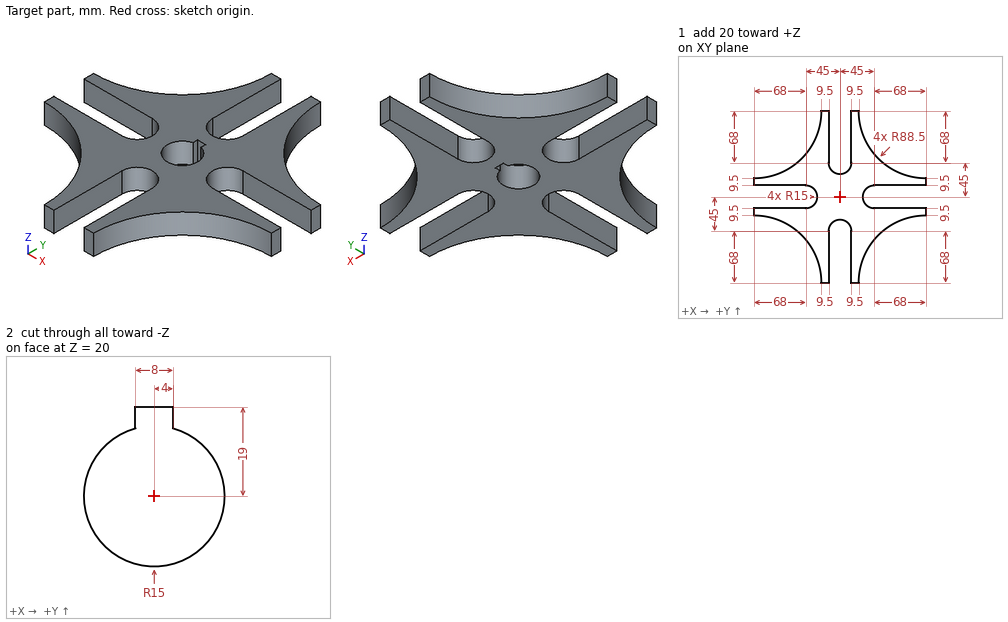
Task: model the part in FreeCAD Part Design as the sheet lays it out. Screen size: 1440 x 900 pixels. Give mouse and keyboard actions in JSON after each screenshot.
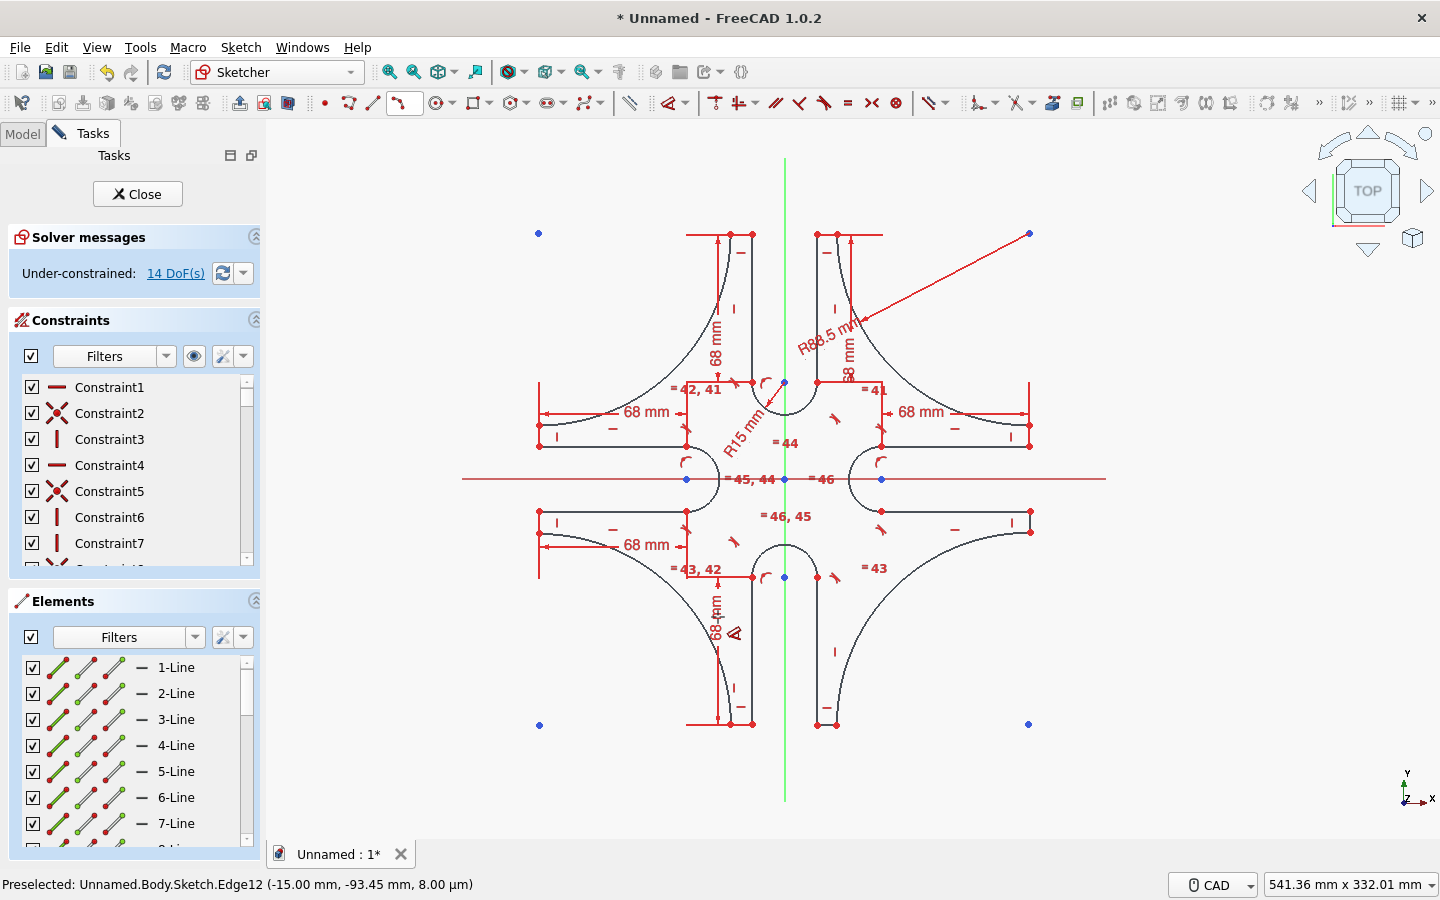
{"action": "left_click", "coordinate": [817, 622]}
{"action": "left_click", "coordinate": [851, 617]}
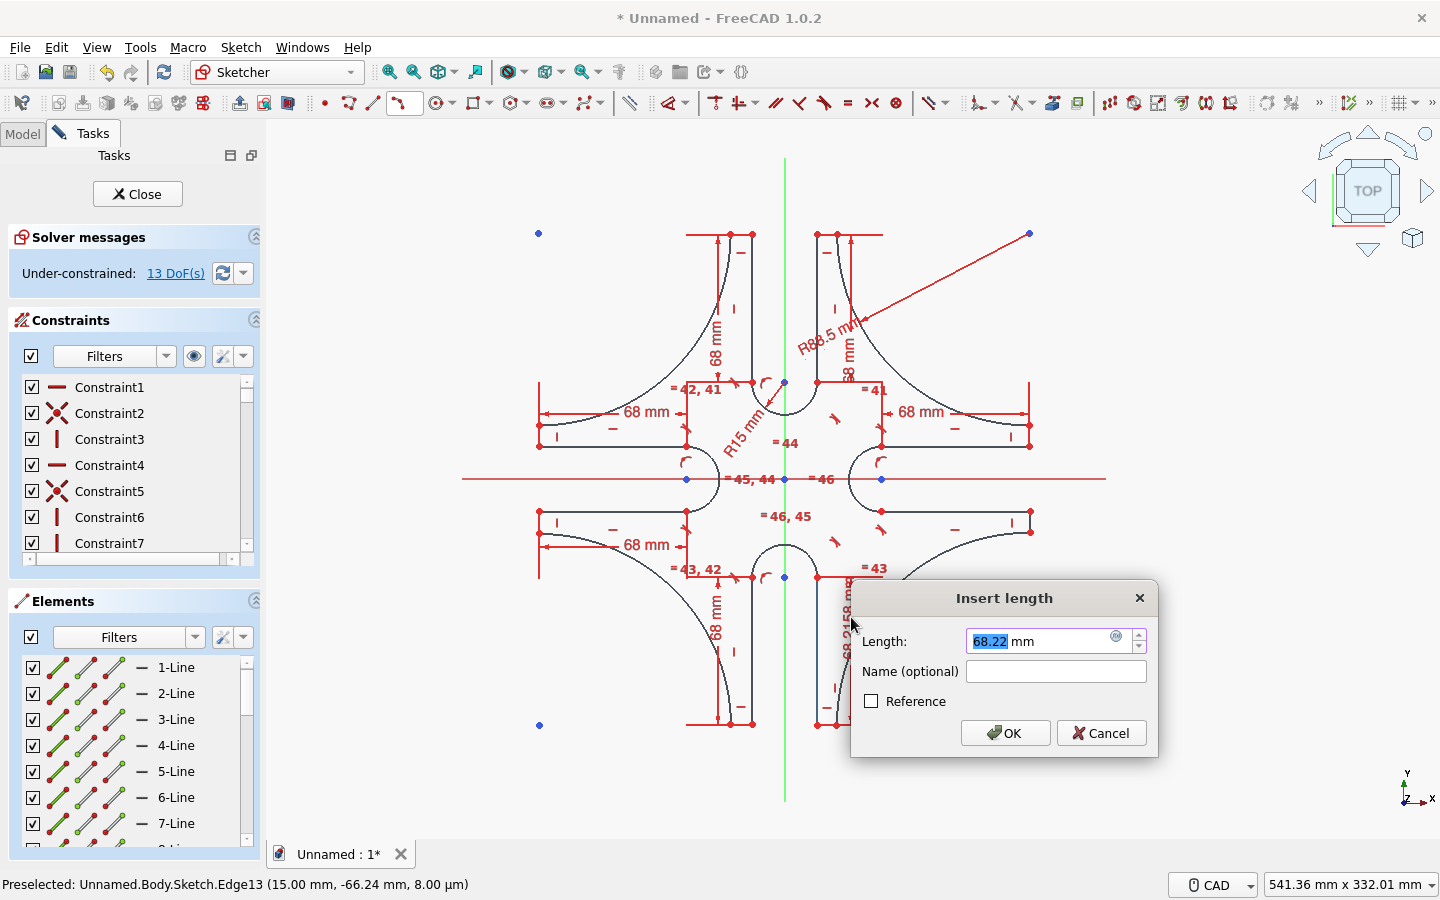
{"action": "type", "text": "68"}
{"action": "key", "text": "Return"}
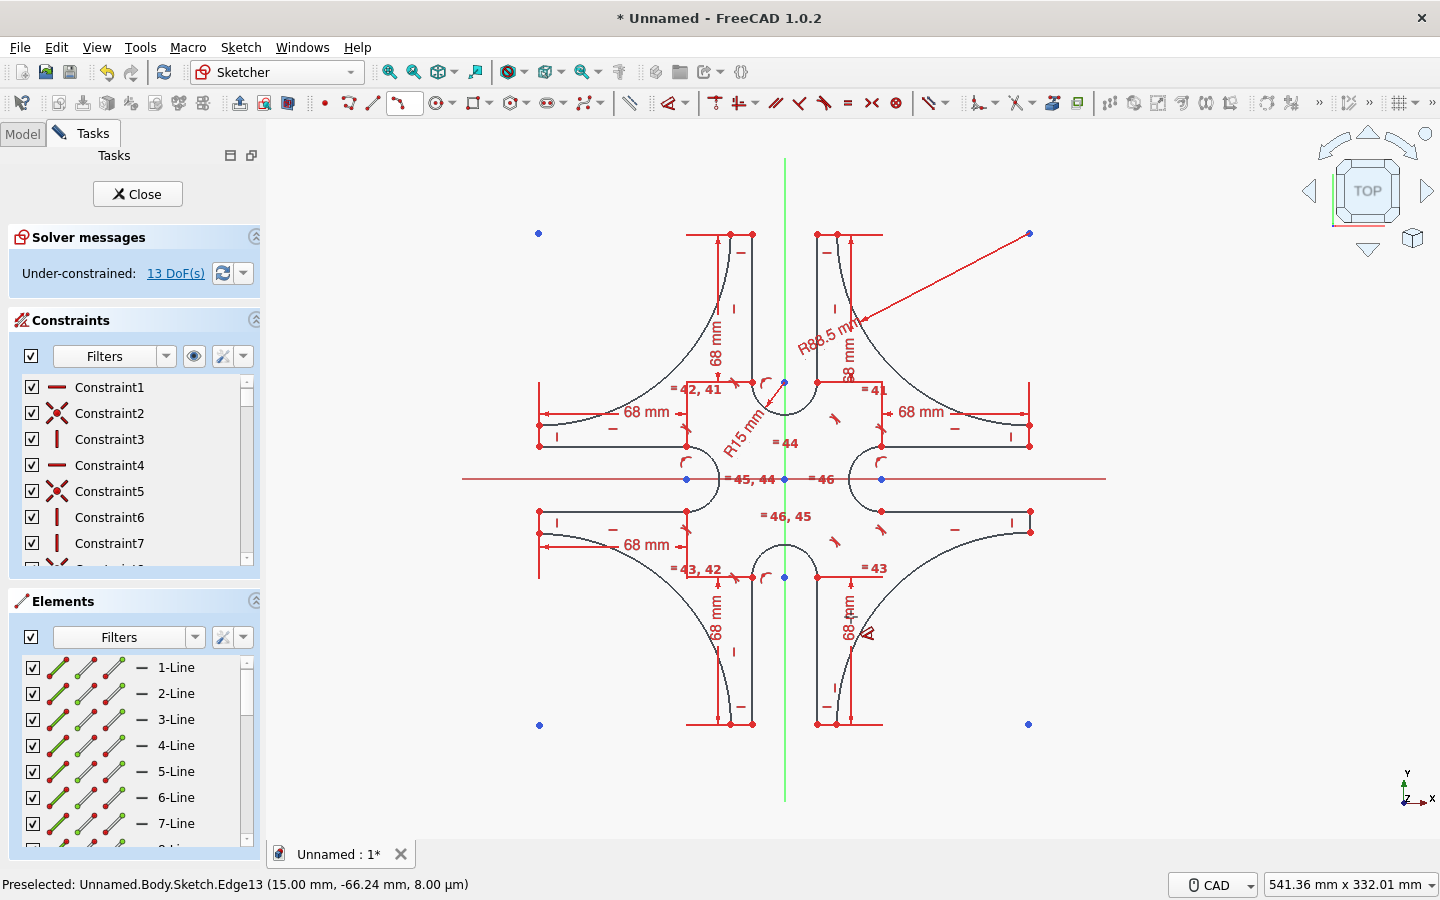
{"action": "left_click", "coordinate": [986, 512]}
{"action": "left_click", "coordinate": [922, 546]}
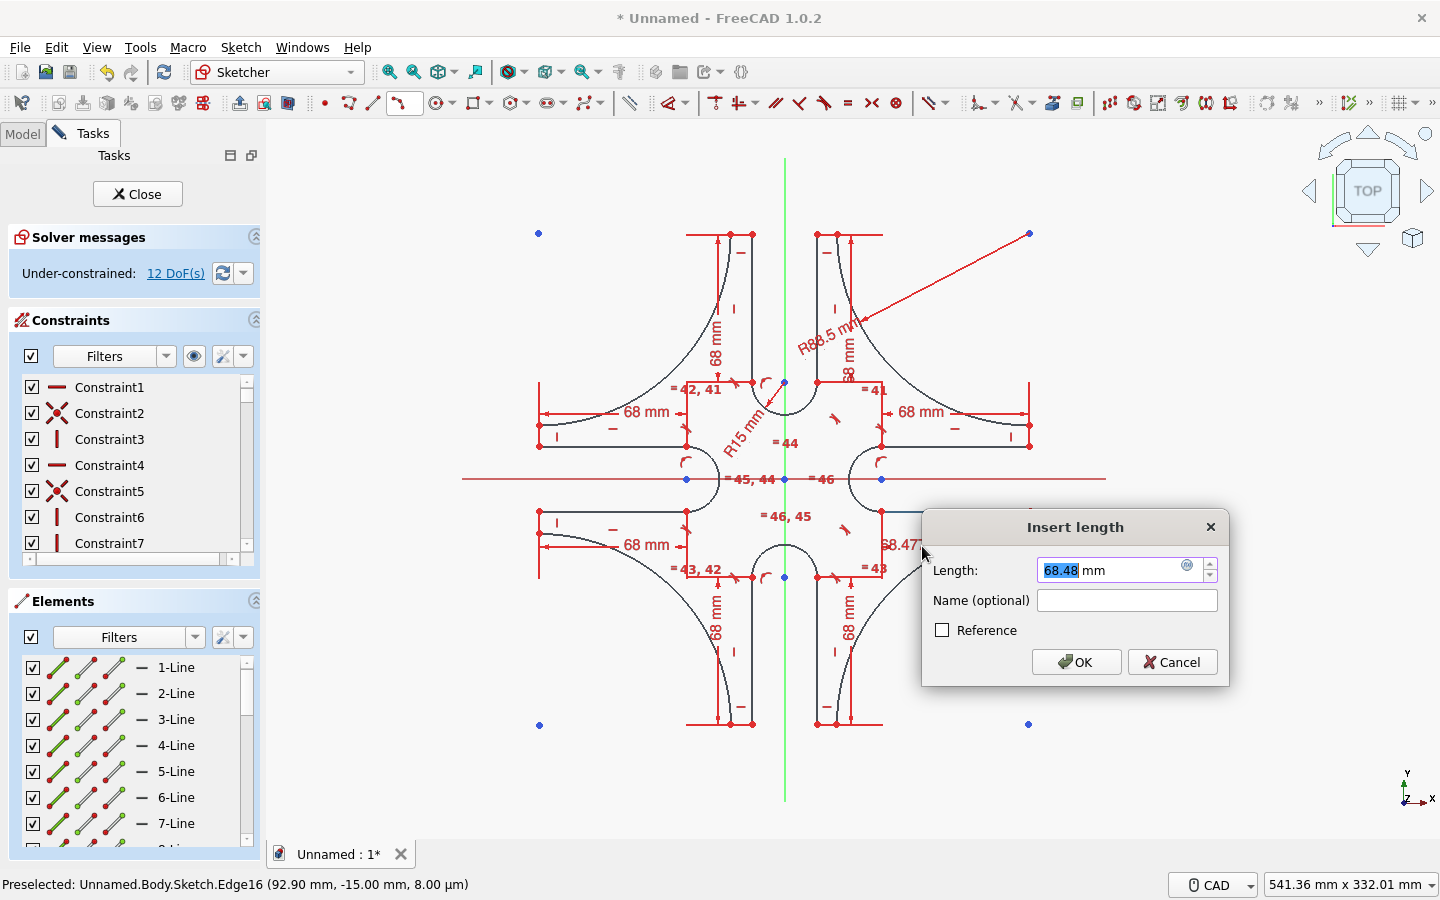
{"action": "type", "text": "68"}
{"action": "key", "text": "Return"}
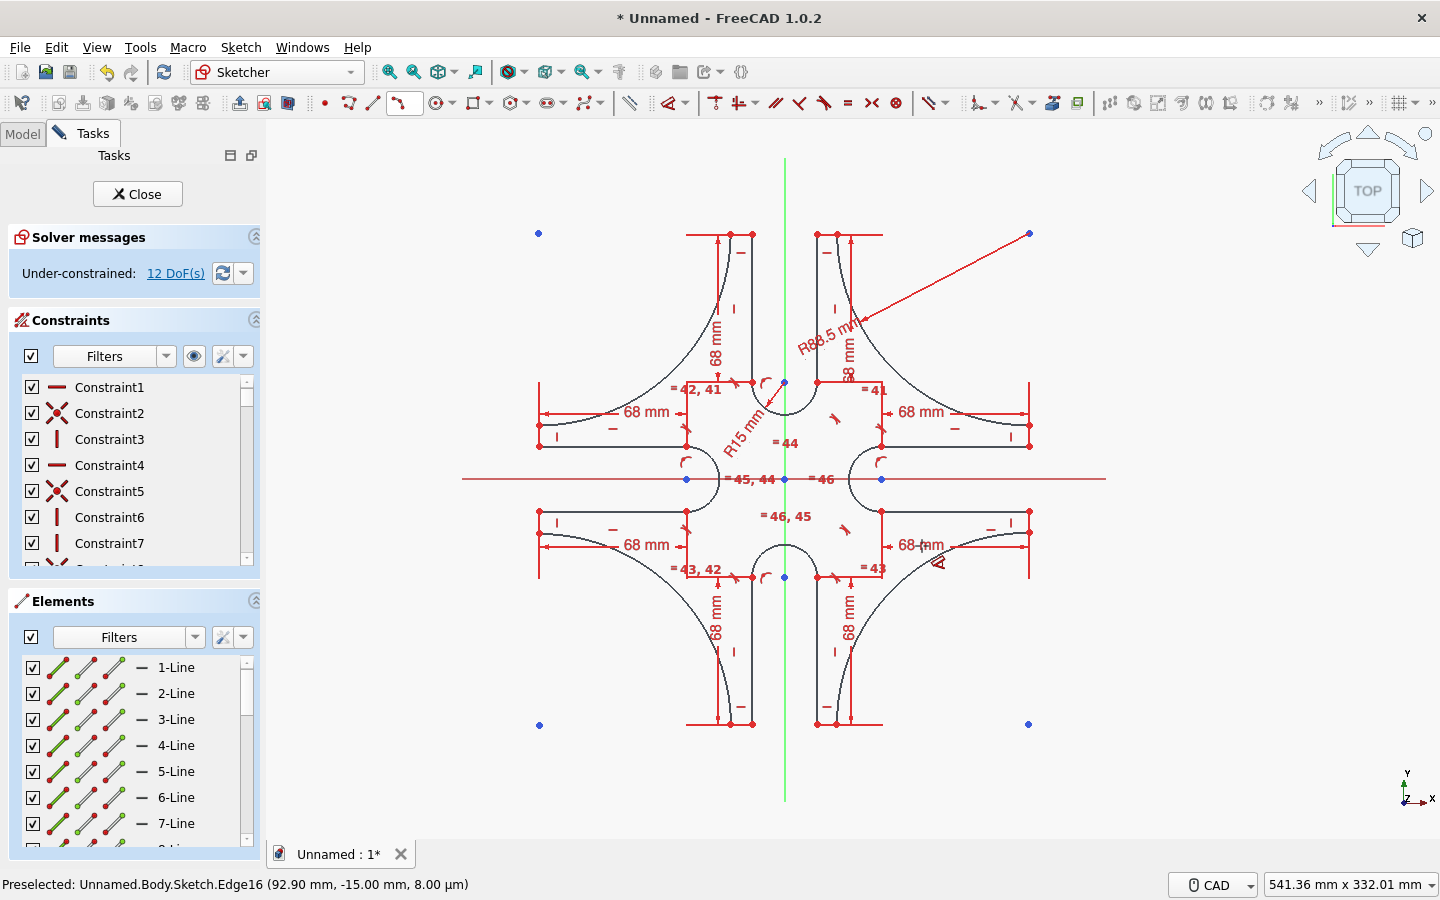
{"action": "scroll", "coordinate": [1029, 436], "scroll_direction": "up", "scroll_amount": 4}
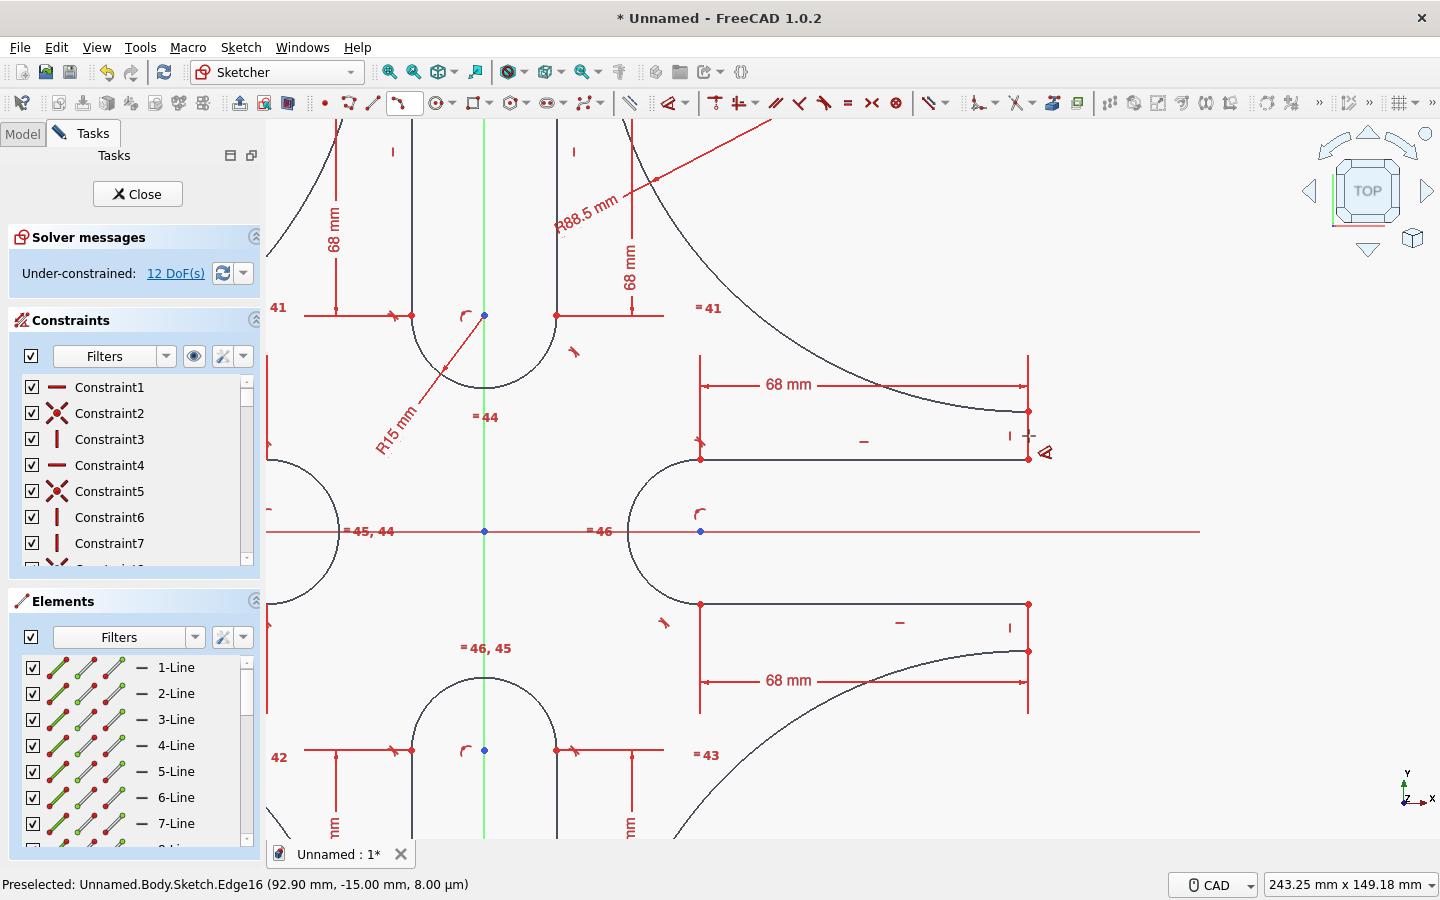
{"action": "left_click", "coordinate": [1028, 436]}
{"action": "left_click", "coordinate": [1062, 436]}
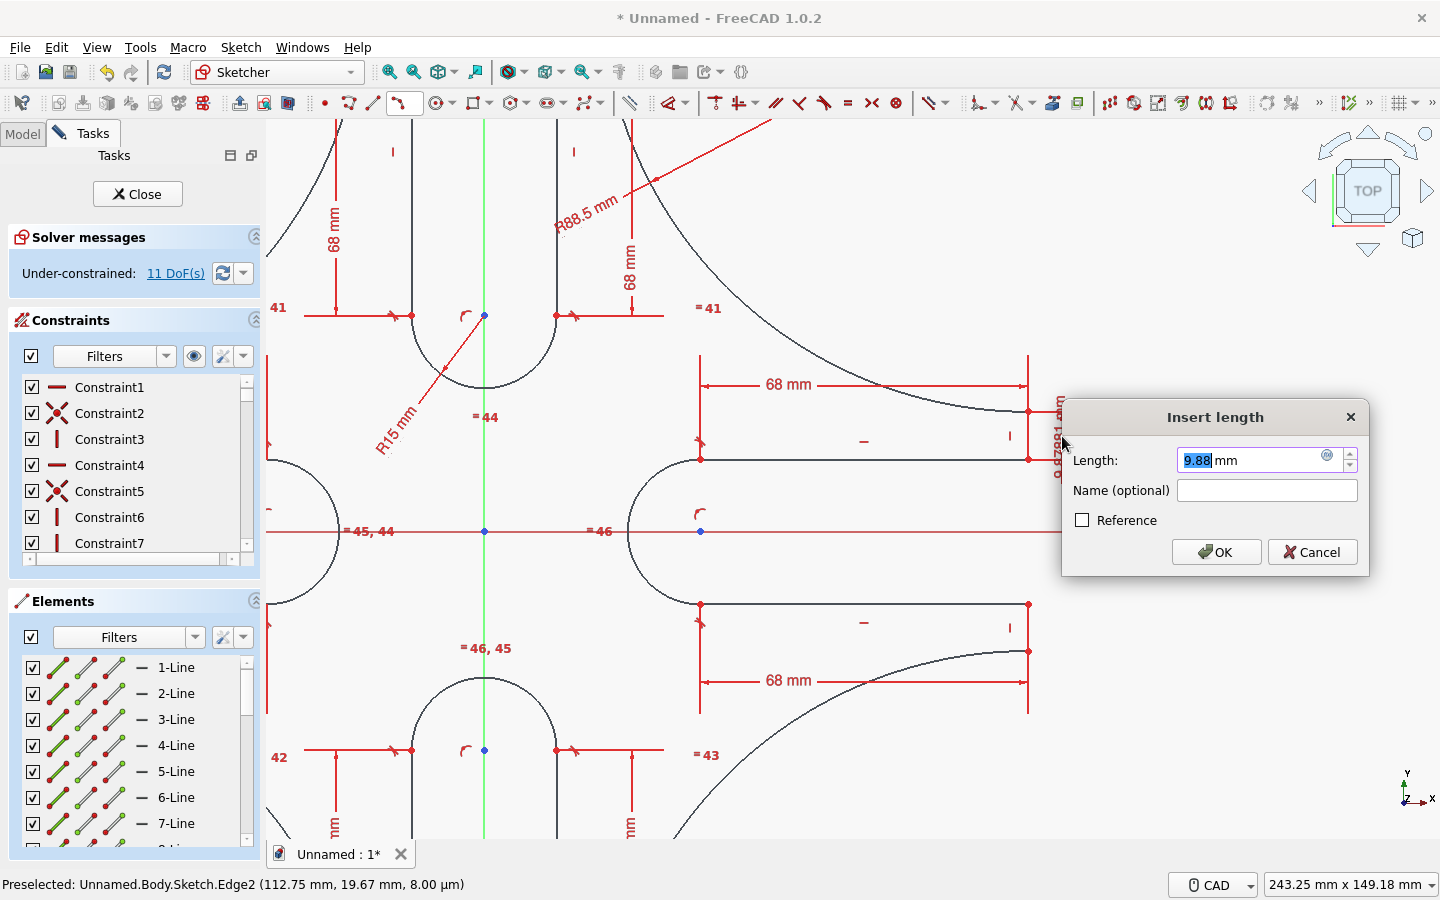
{"action": "type", "text": "9.5"}
{"action": "key", "text": "Return"}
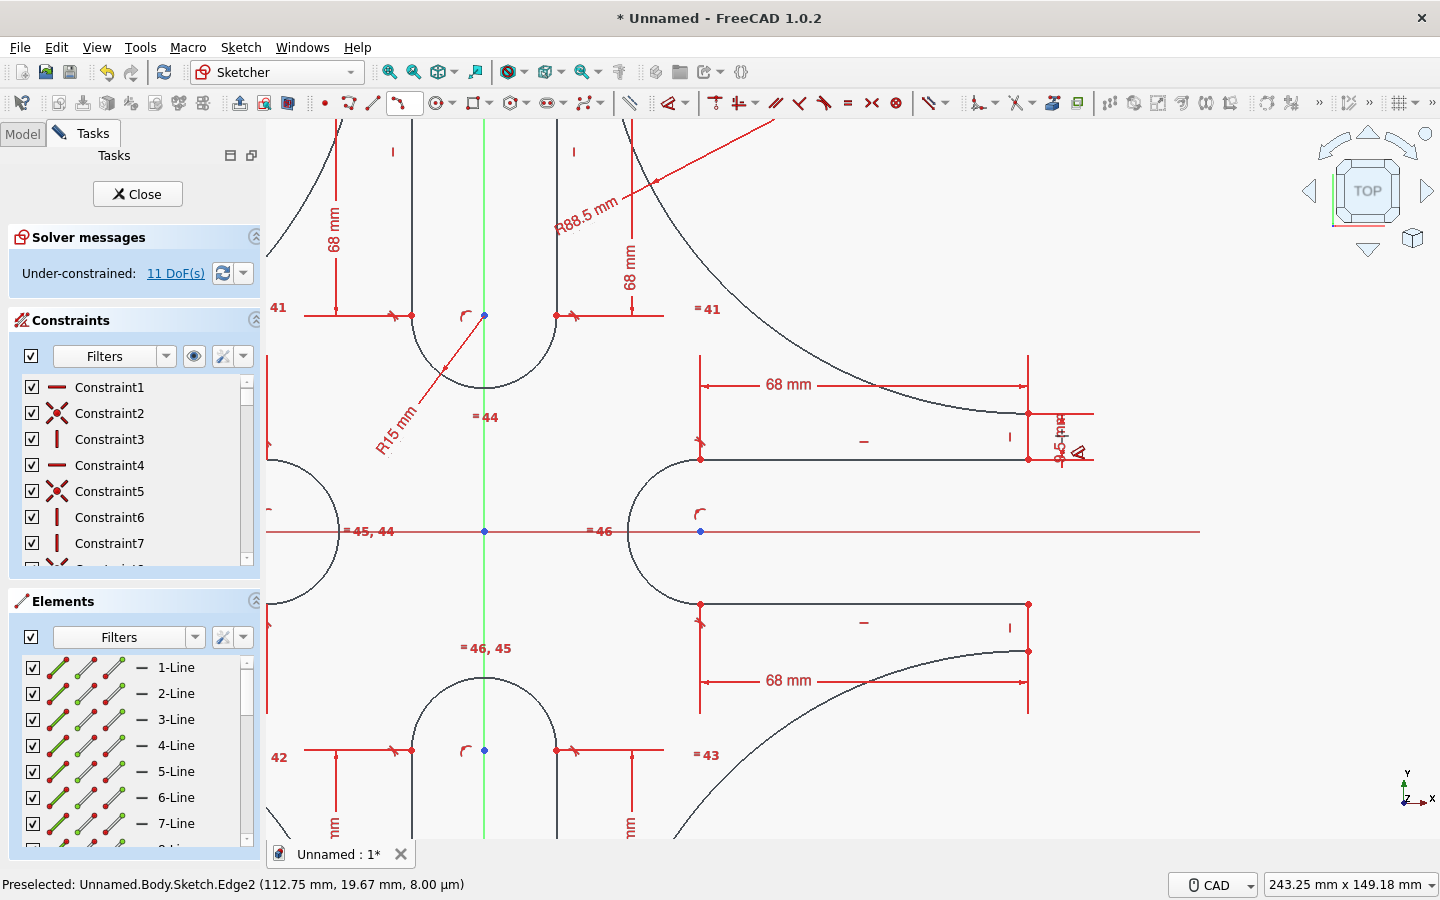
{"action": "scroll", "coordinate": [1030, 436], "scroll_direction": "down", "scroll_amount": 4}